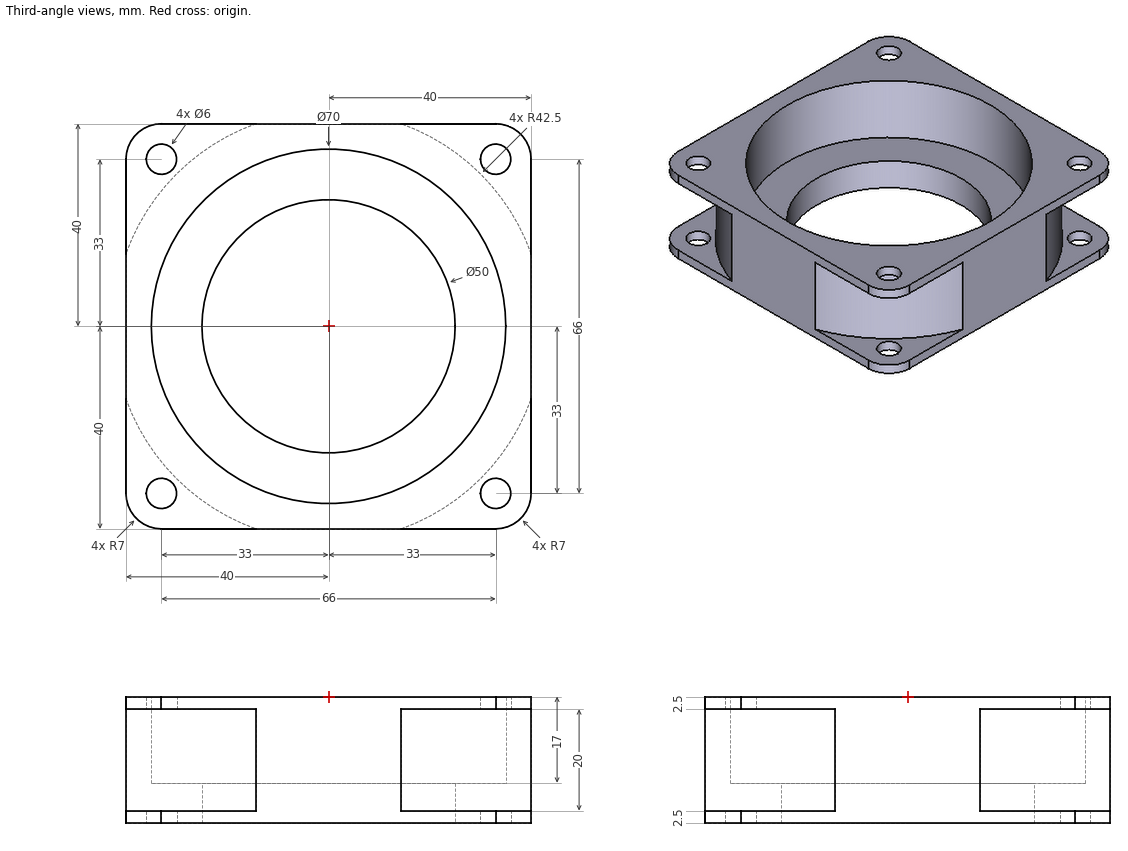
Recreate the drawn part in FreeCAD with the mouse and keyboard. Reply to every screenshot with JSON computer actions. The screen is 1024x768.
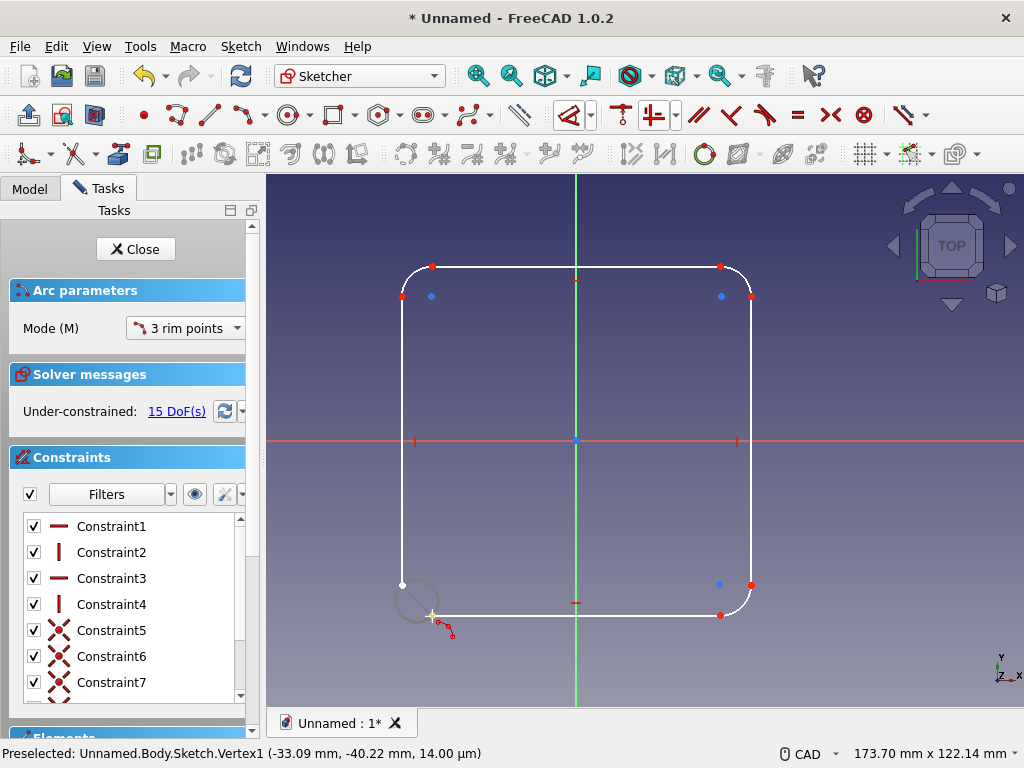
{"action": "scroll", "coordinate": [411, 606], "scroll_direction": "up", "scroll_amount": 3}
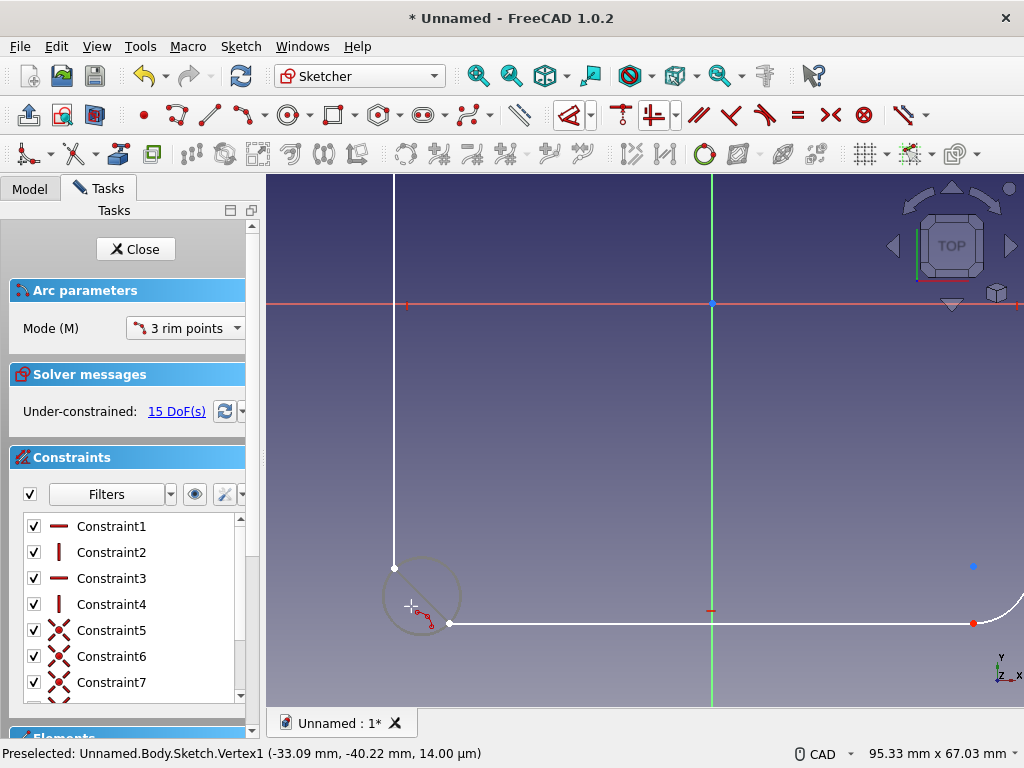
{"action": "left_click", "coordinate": [410, 606]}
{"action": "key", "text": "Escape"}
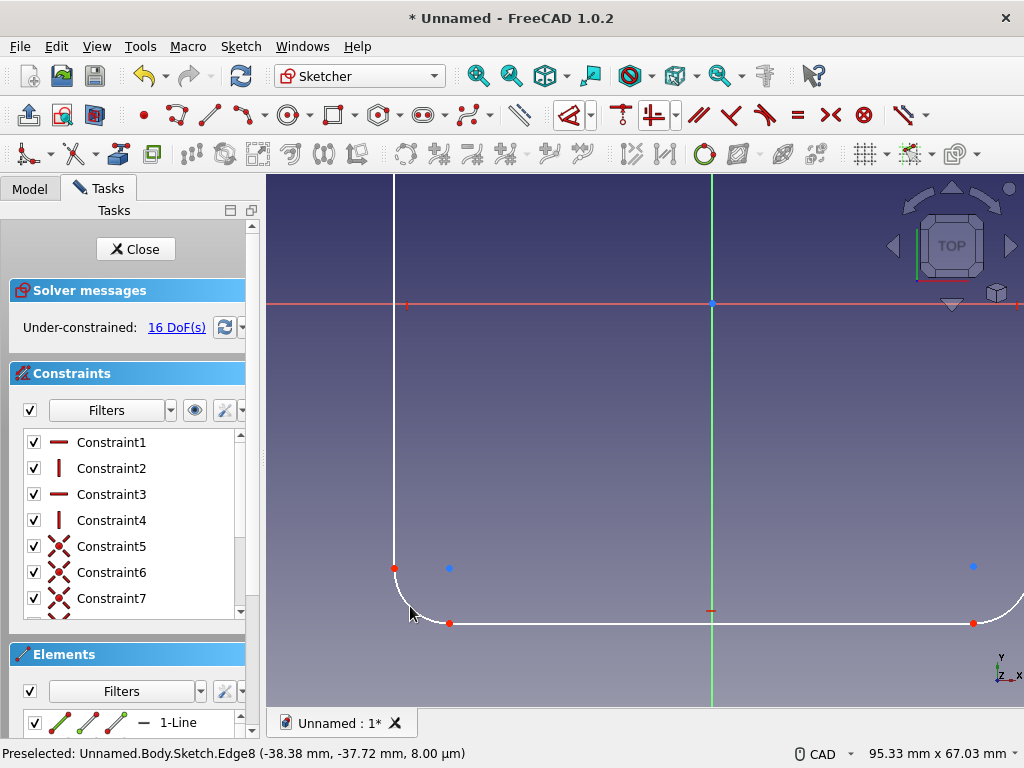
{"action": "left_click", "coordinate": [607, 624]}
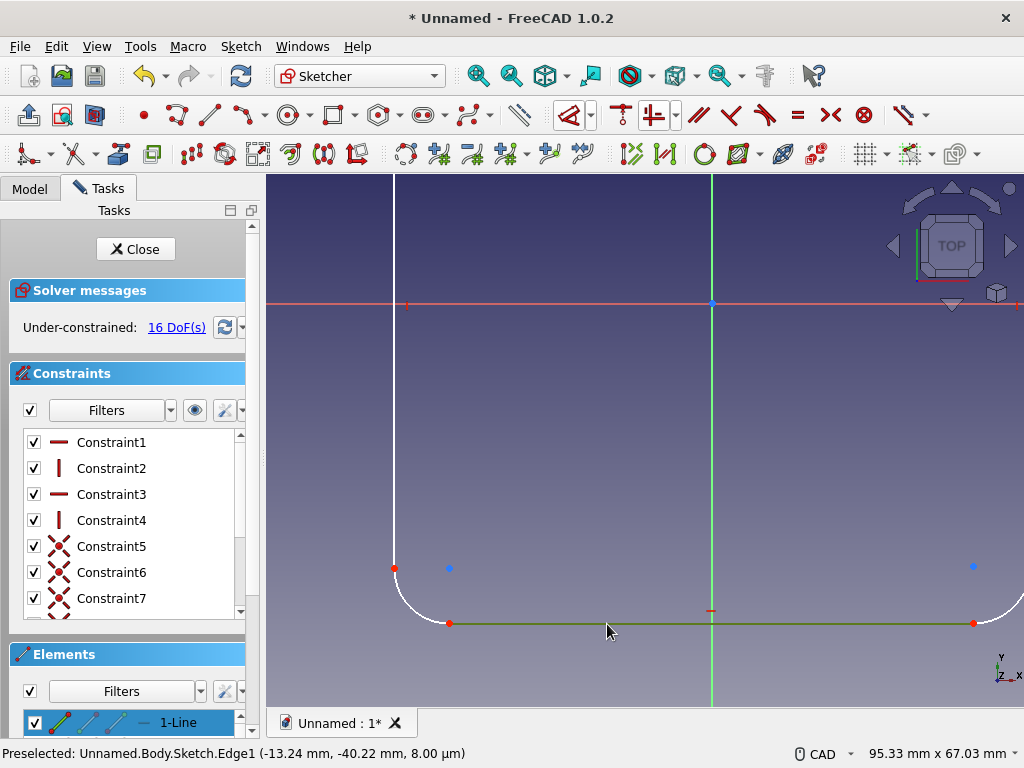
{"action": "scroll", "coordinate": [411, 607], "scroll_direction": "down", "scroll_amount": 3}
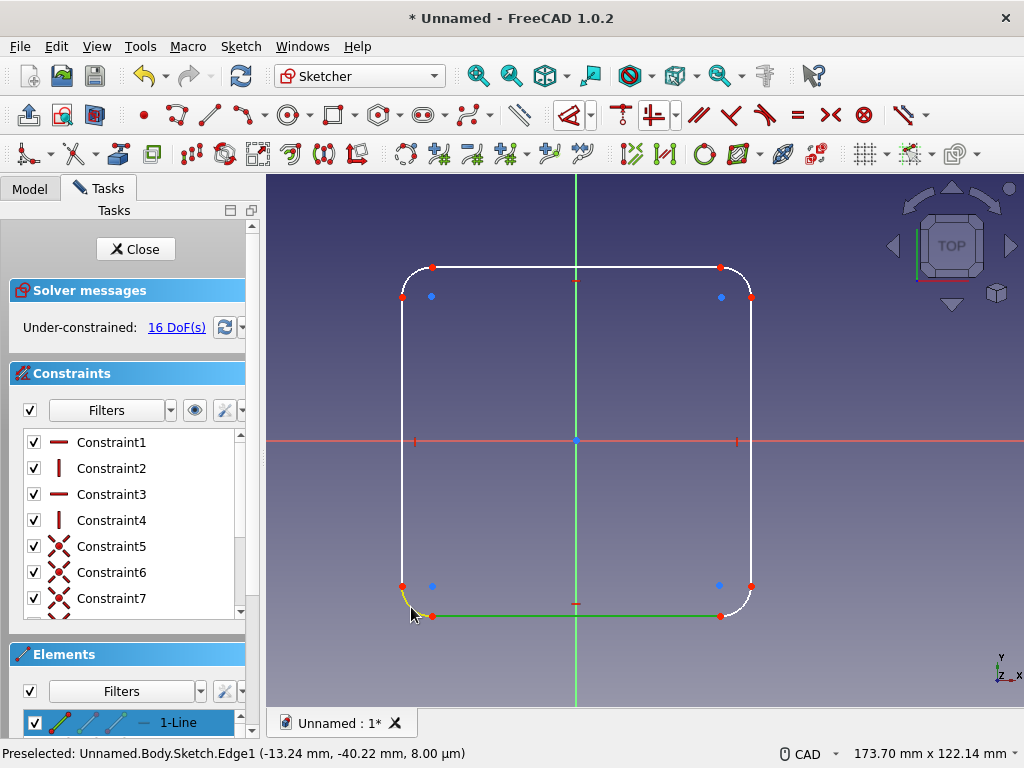
{"action": "left_click", "coordinate": [734, 613]}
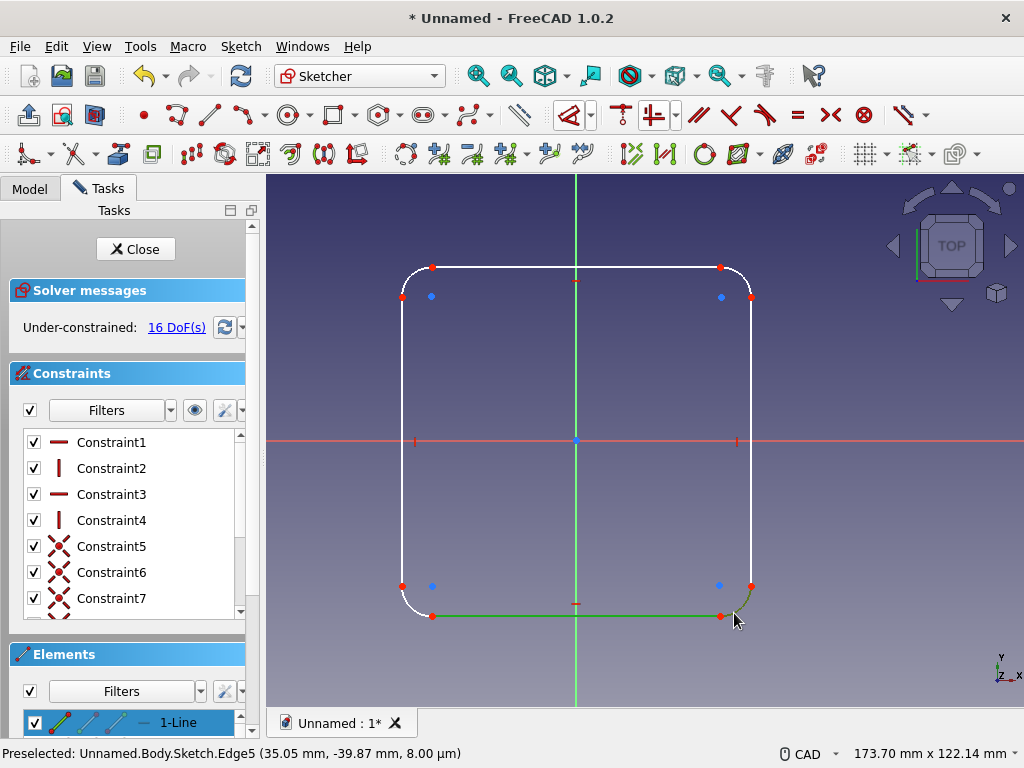
{"action": "left_click", "coordinate": [765, 116]}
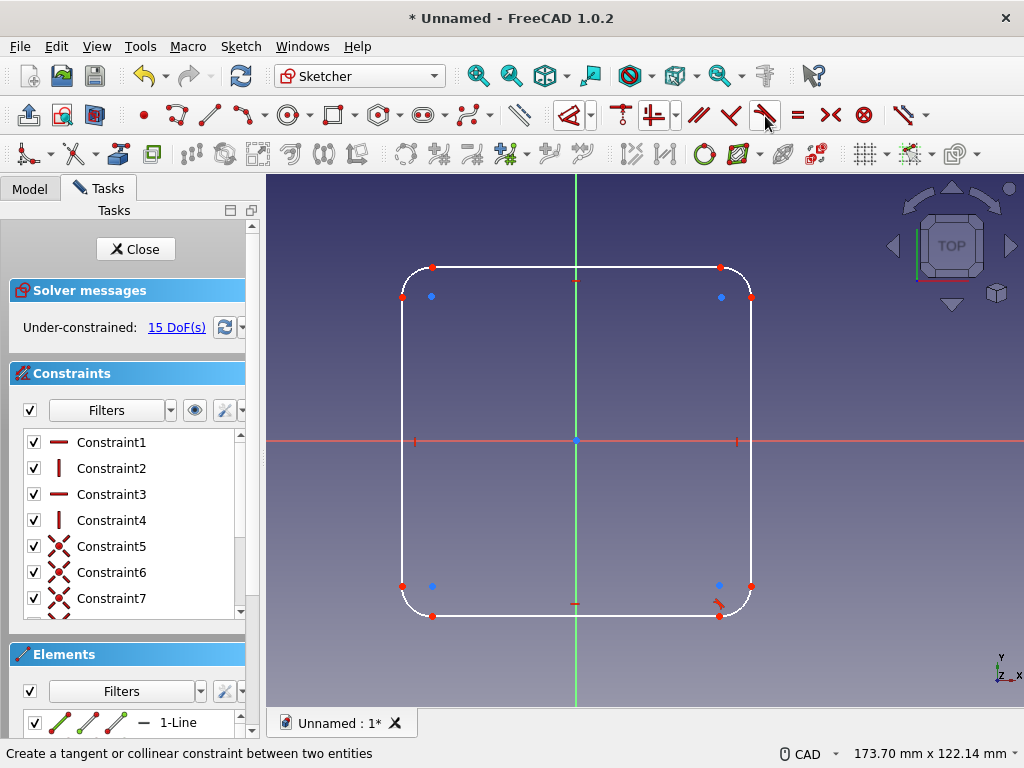
{"action": "left_click", "coordinate": [518, 616]}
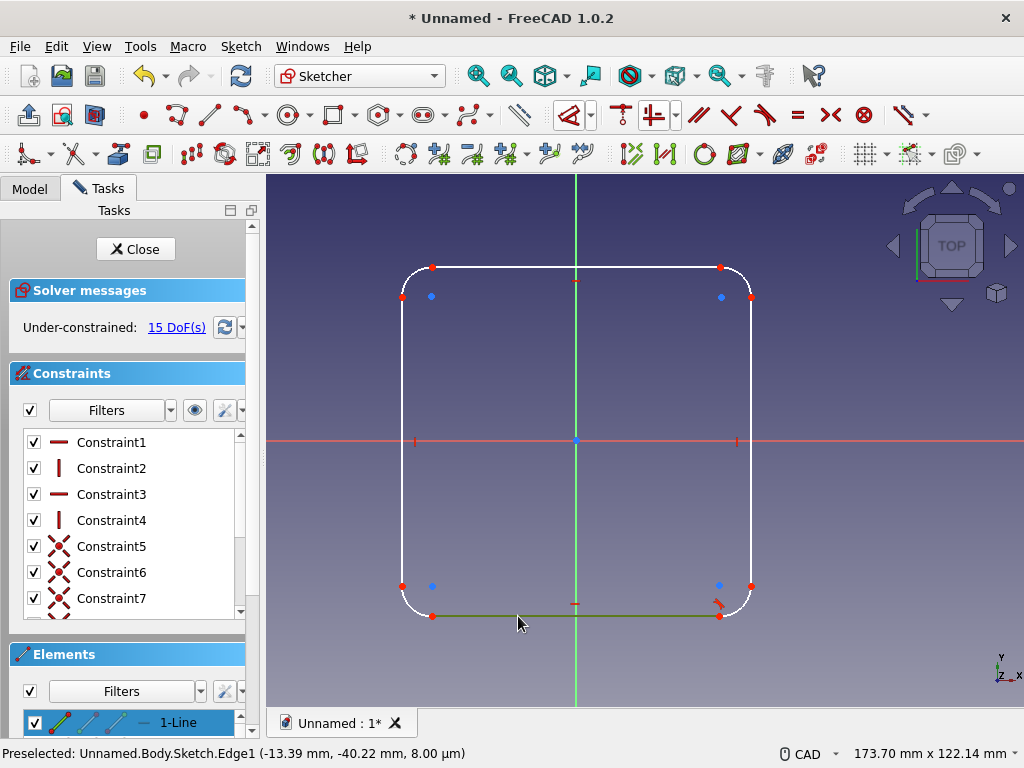
{"action": "left_click", "coordinate": [405, 600]}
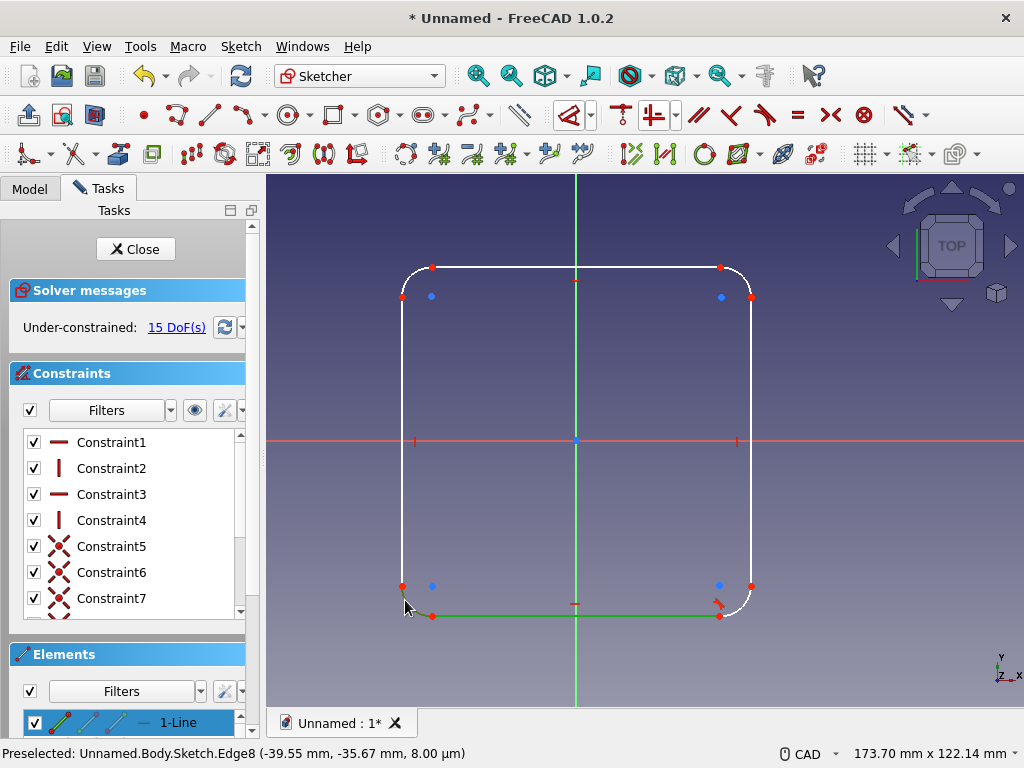
{"action": "left_click", "coordinate": [765, 116]}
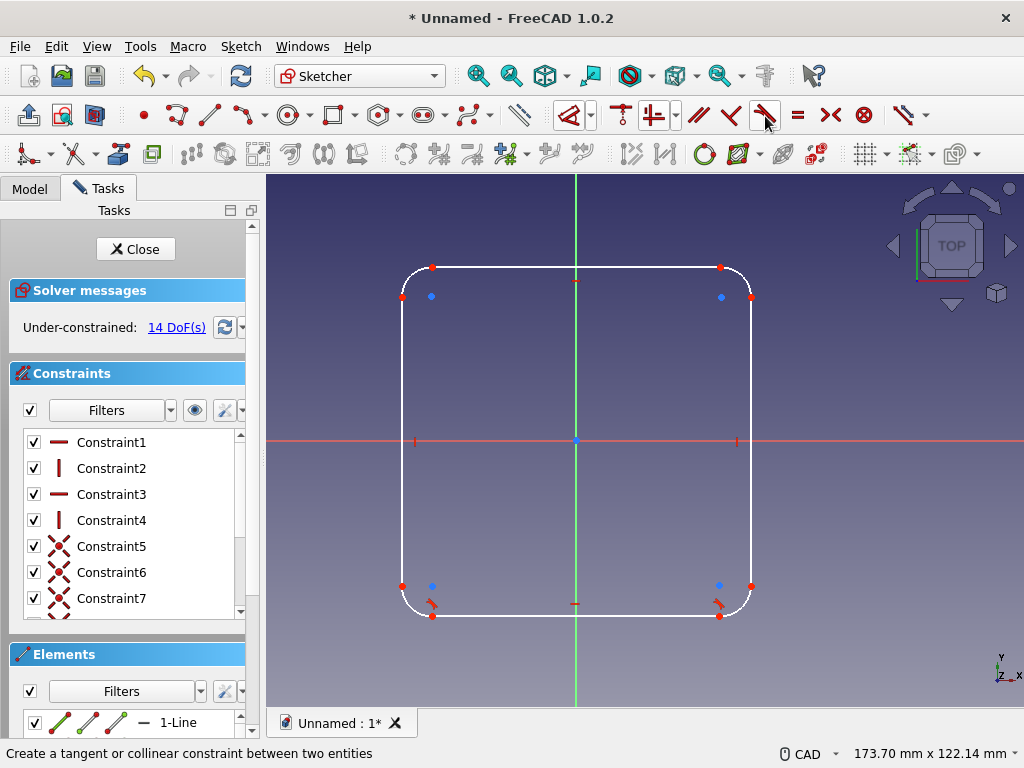
{"action": "left_click", "coordinate": [751, 500]}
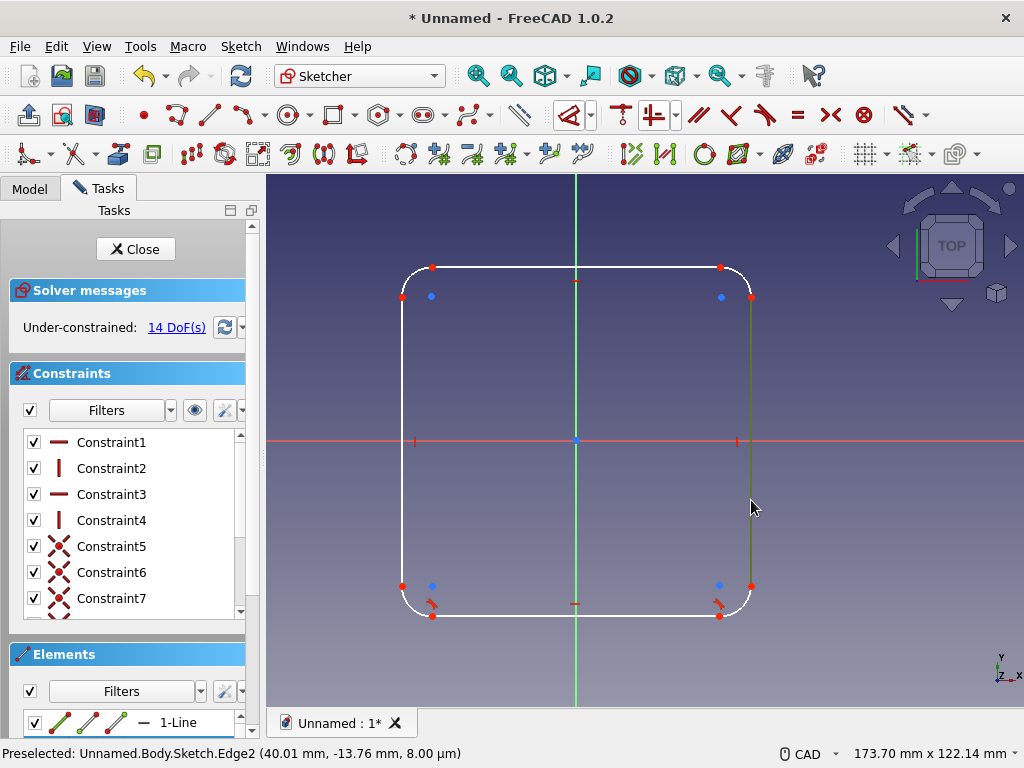
{"action": "left_click", "coordinate": [734, 613]}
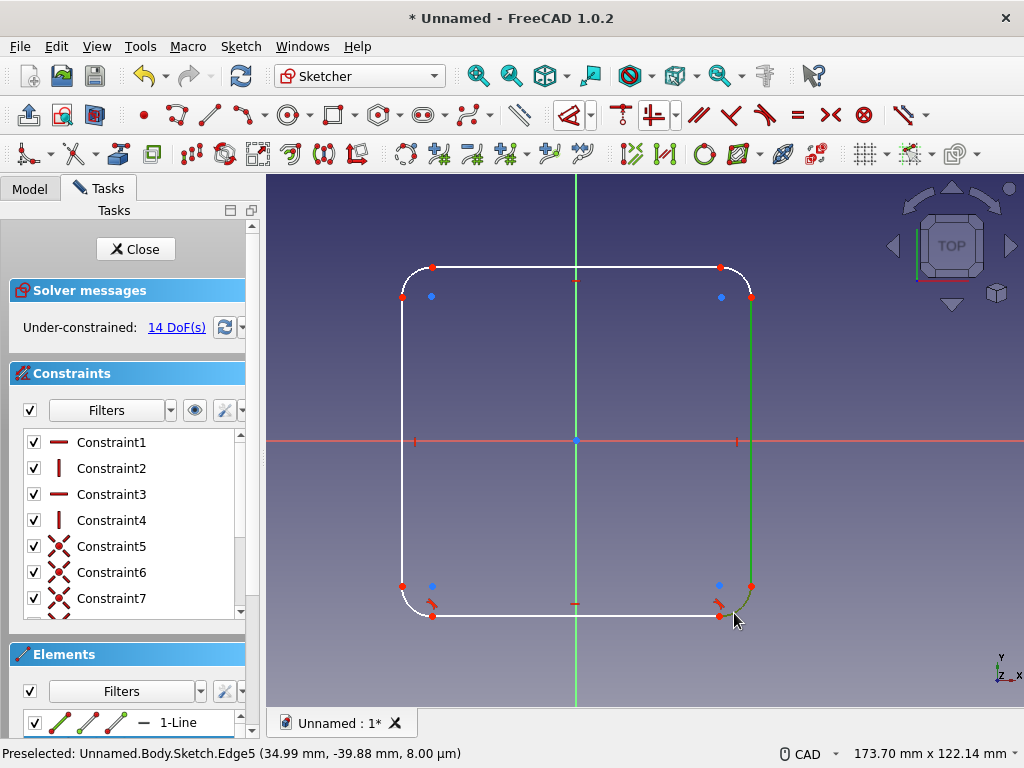
{"action": "left_click", "coordinate": [765, 116]}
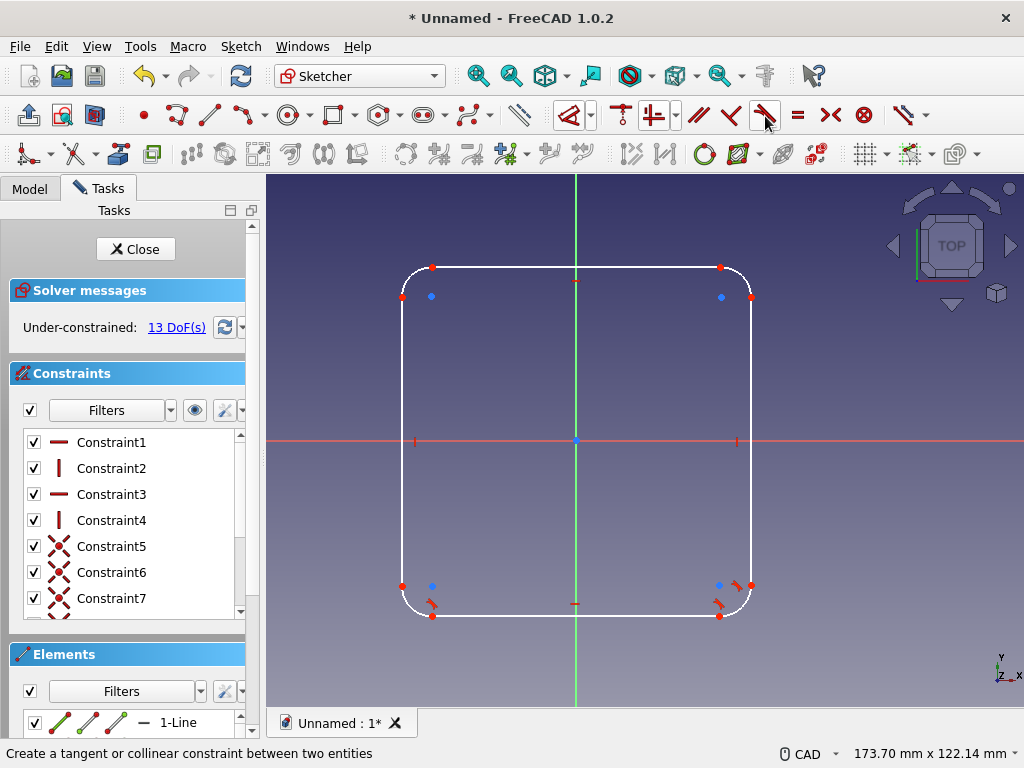
{"action": "left_click", "coordinate": [751, 499]}